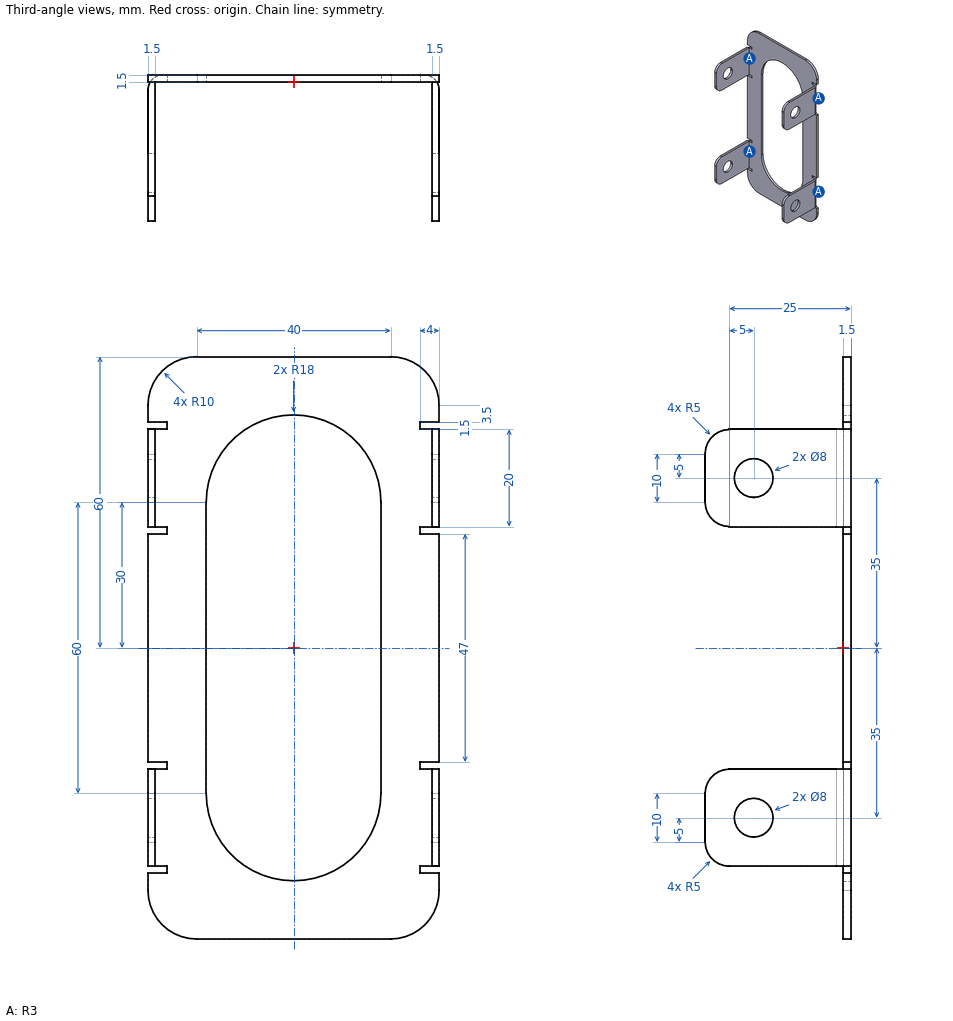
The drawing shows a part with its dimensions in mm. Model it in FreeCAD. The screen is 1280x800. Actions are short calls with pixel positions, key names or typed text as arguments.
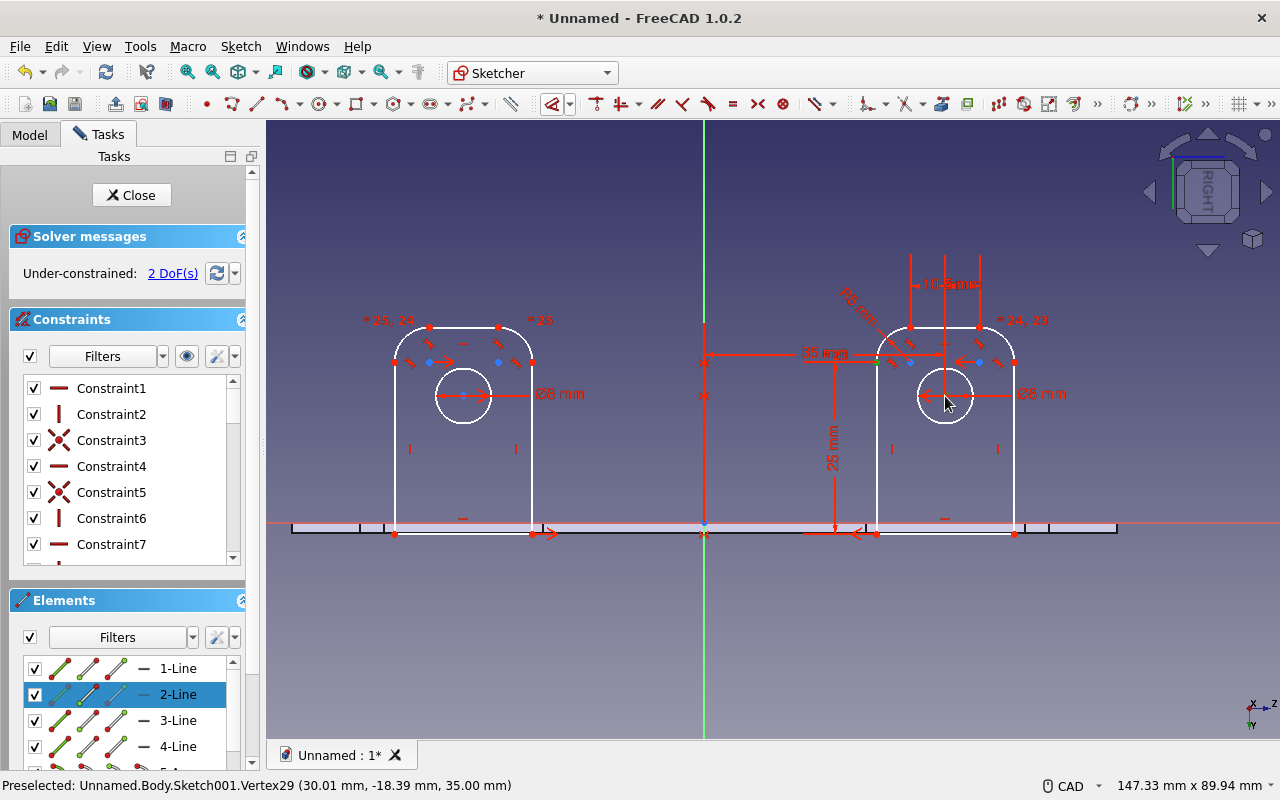
key(i)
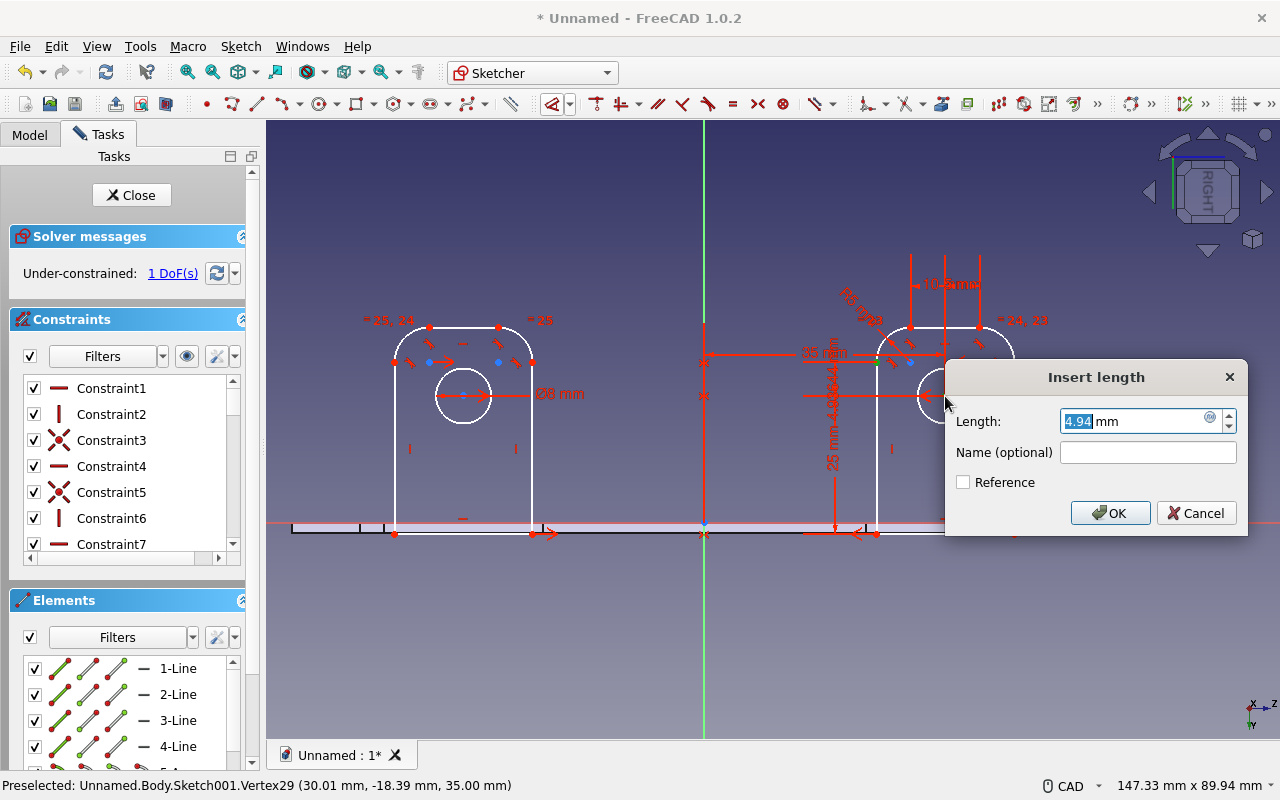
text(5)
key(Return)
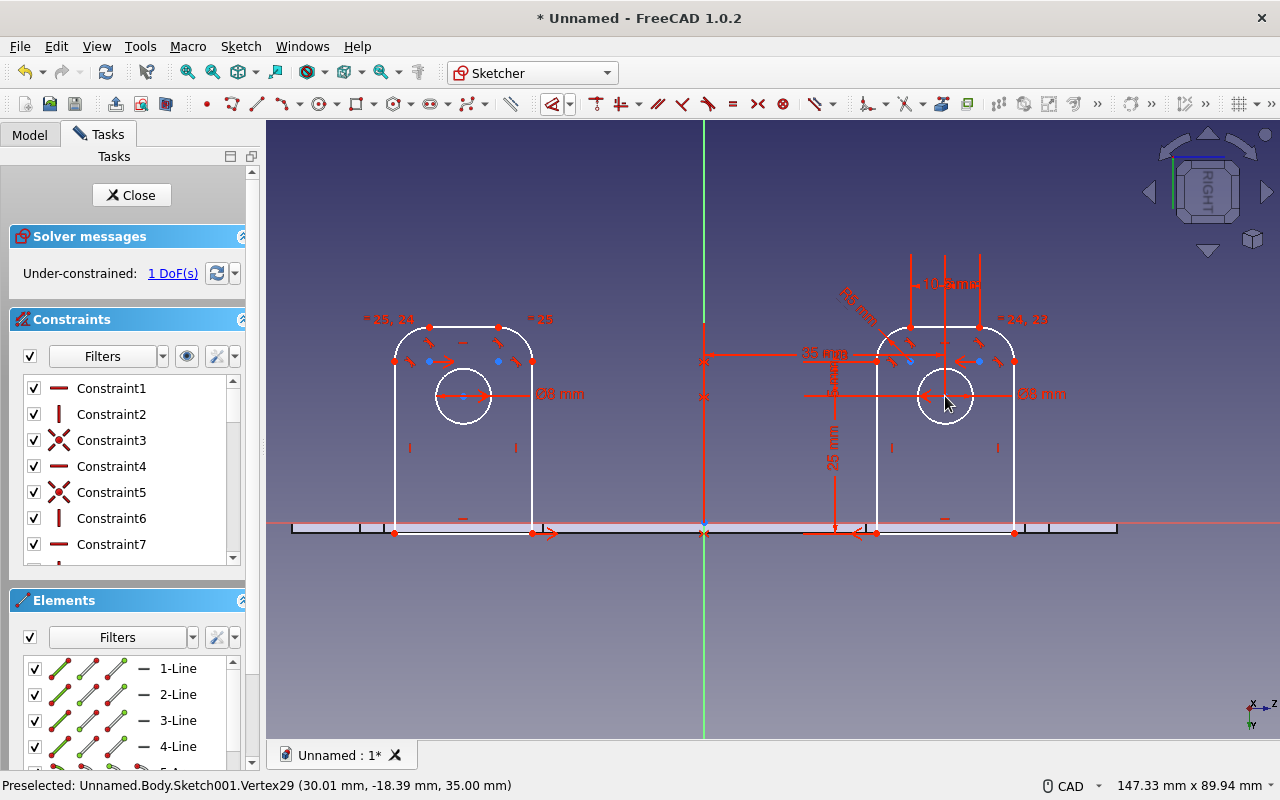
scroll(877, 534, up, 7)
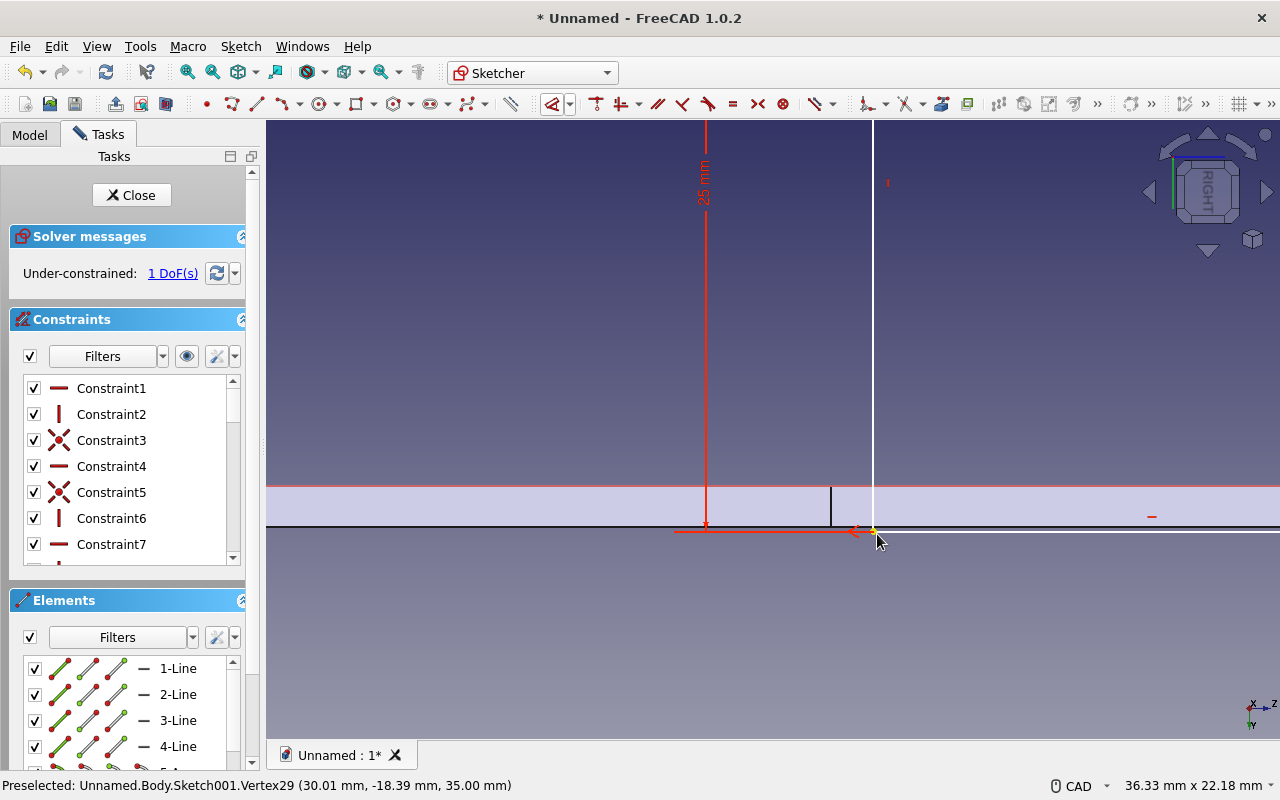
click(873, 532)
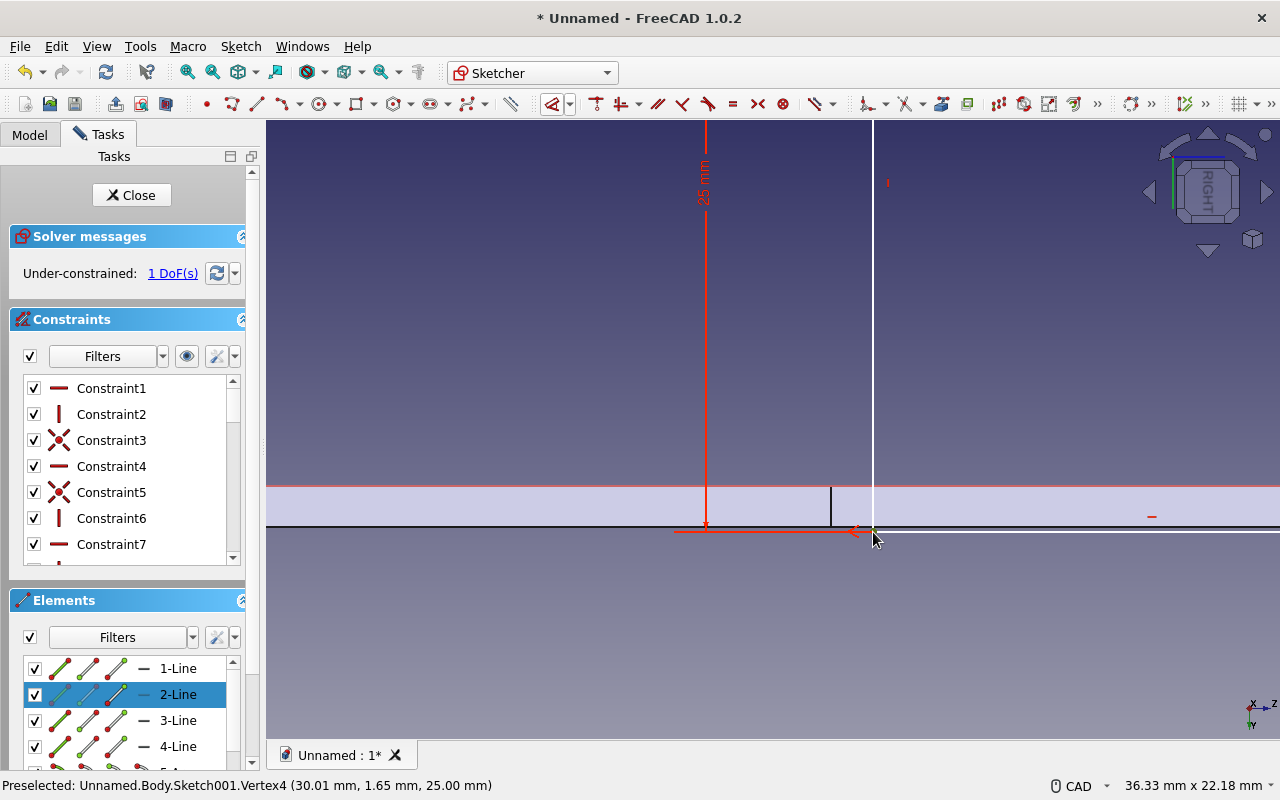
key(i)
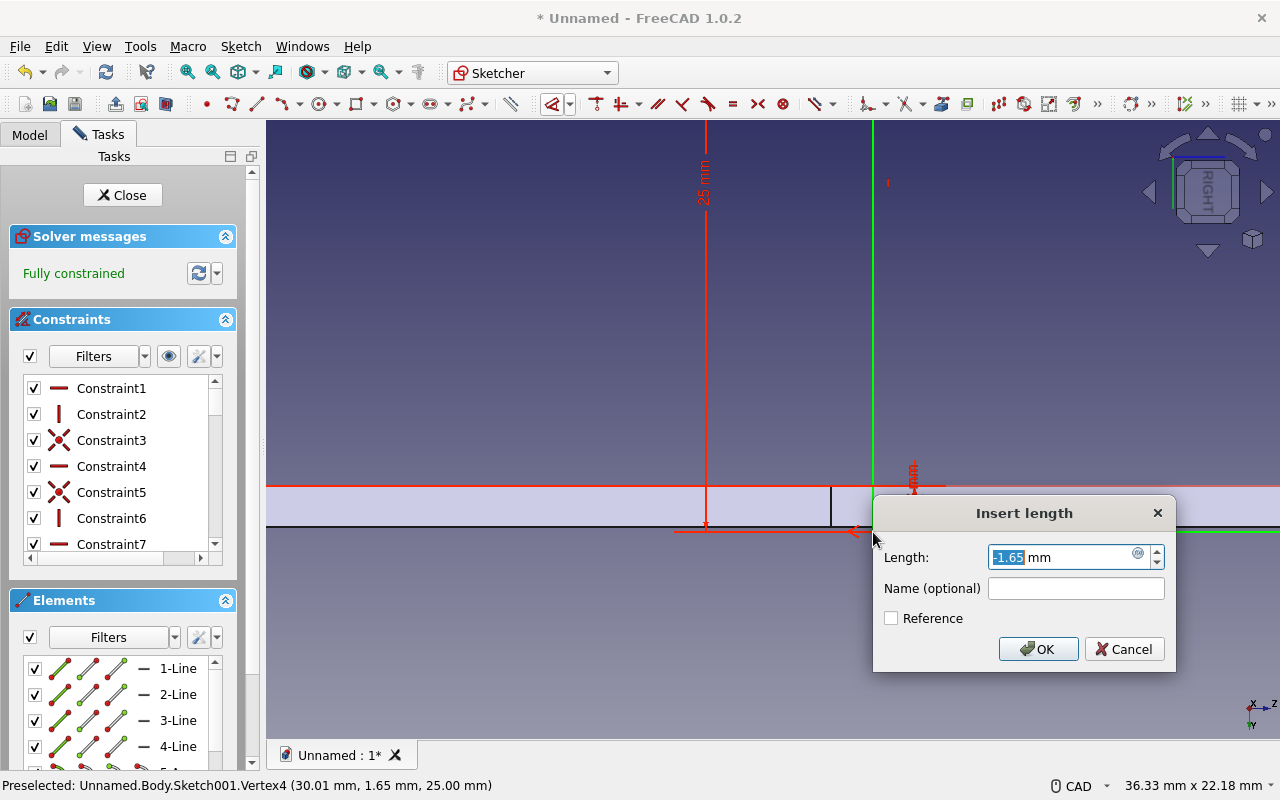
text(-1.5)
key(Return)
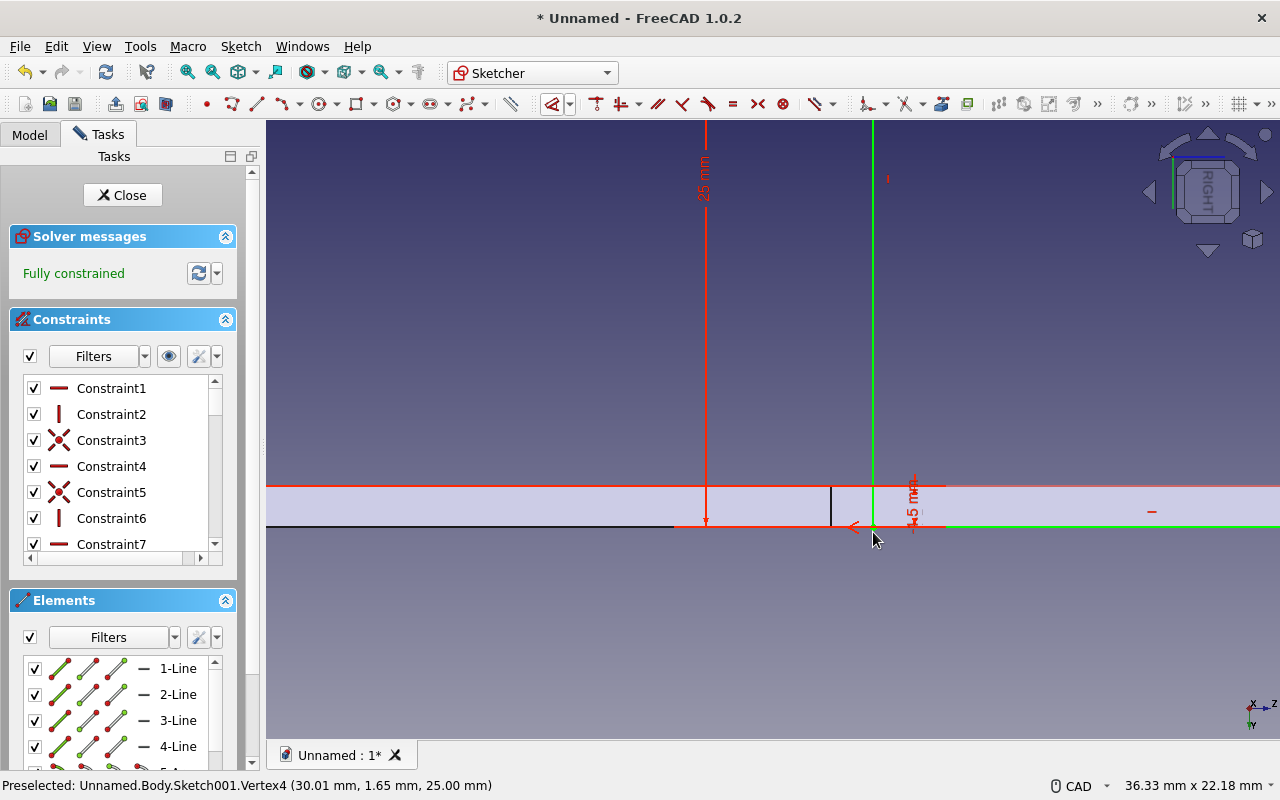
click(123, 195)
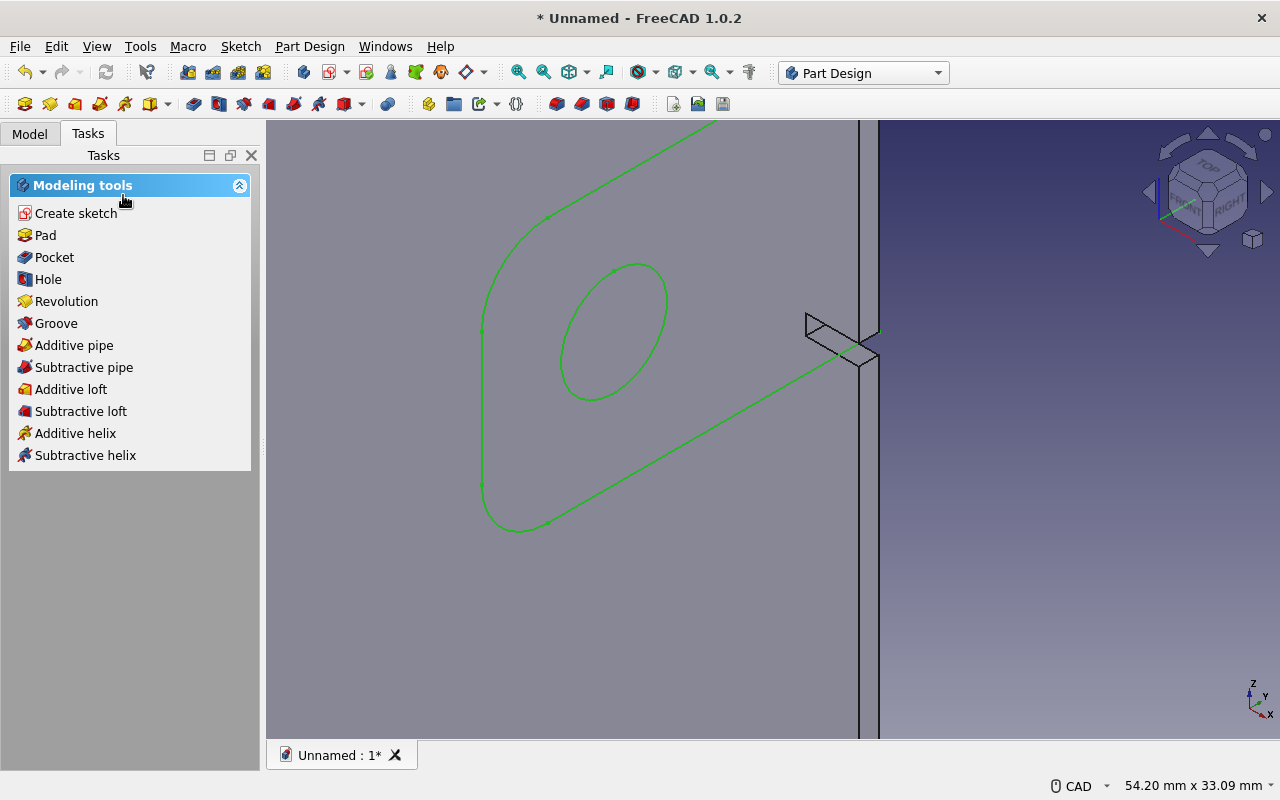
click(25, 104)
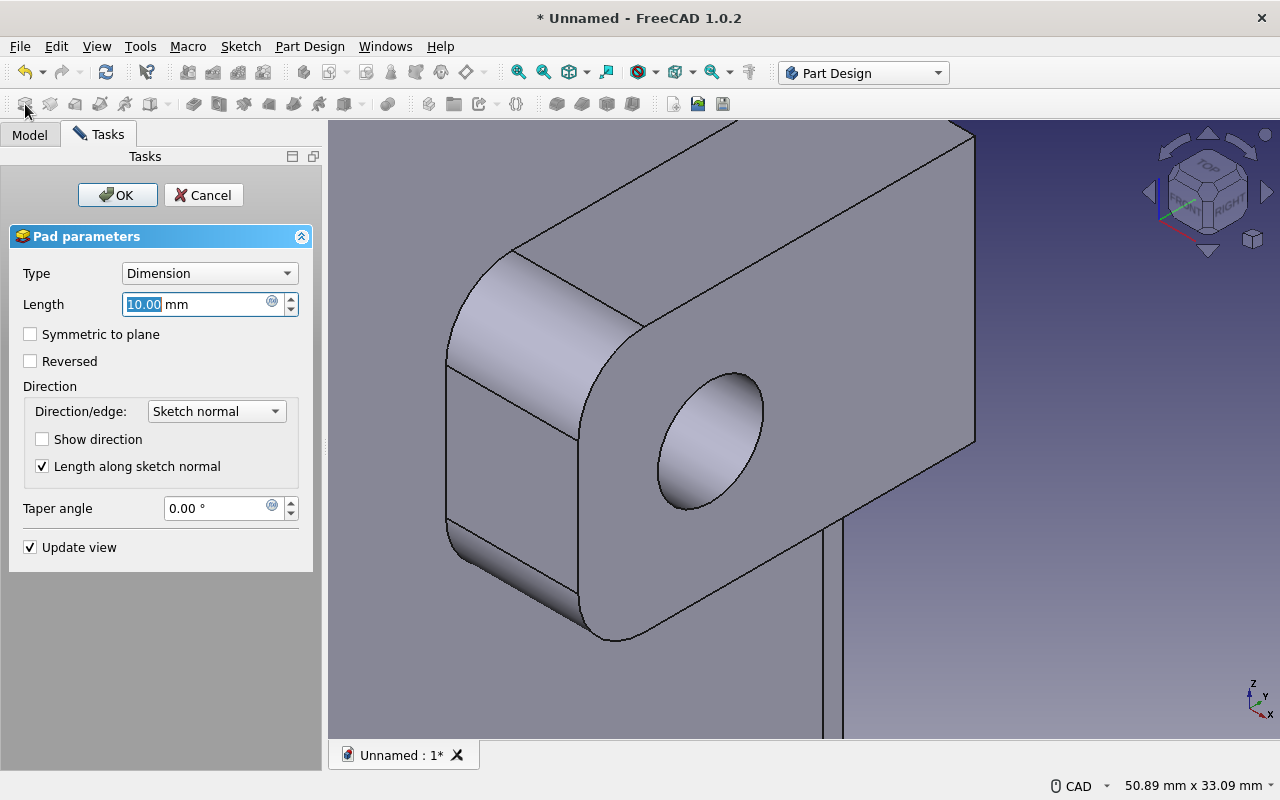
text(1.5)
key(Tab)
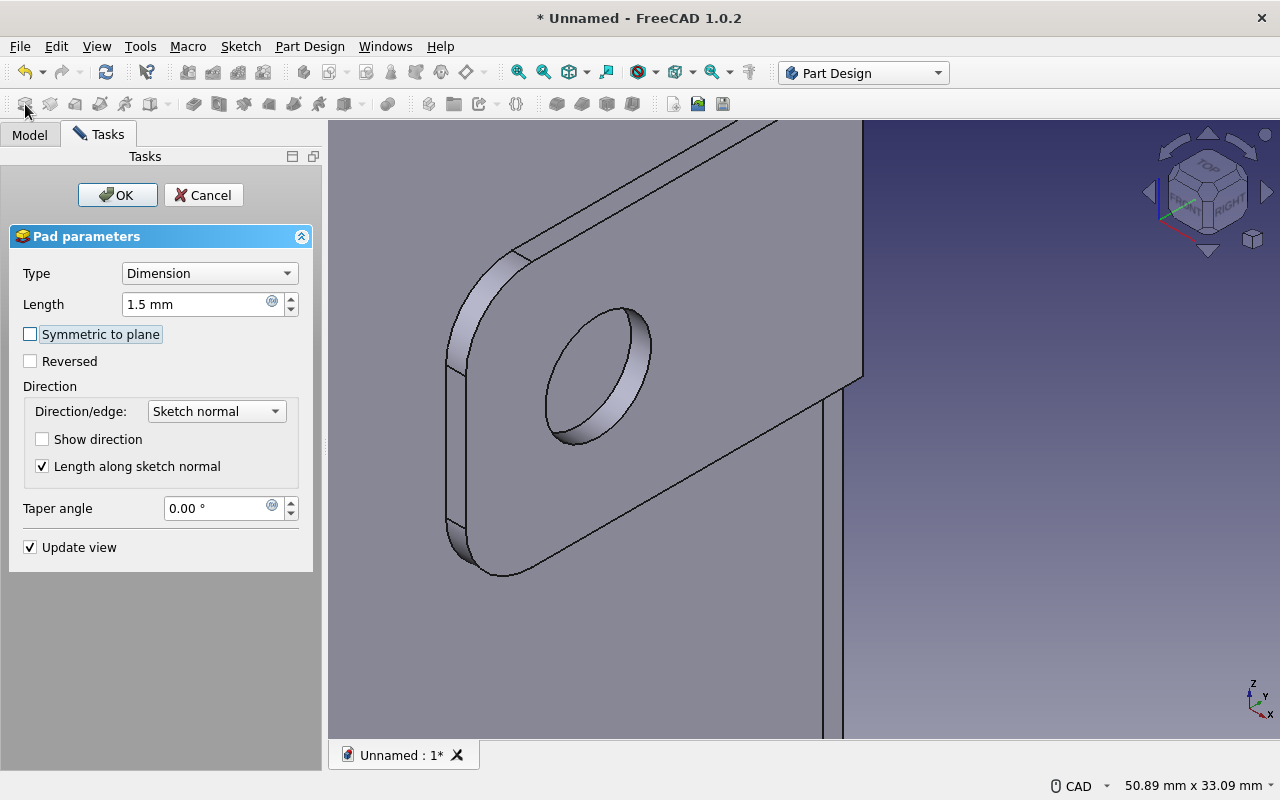
click(31, 361)